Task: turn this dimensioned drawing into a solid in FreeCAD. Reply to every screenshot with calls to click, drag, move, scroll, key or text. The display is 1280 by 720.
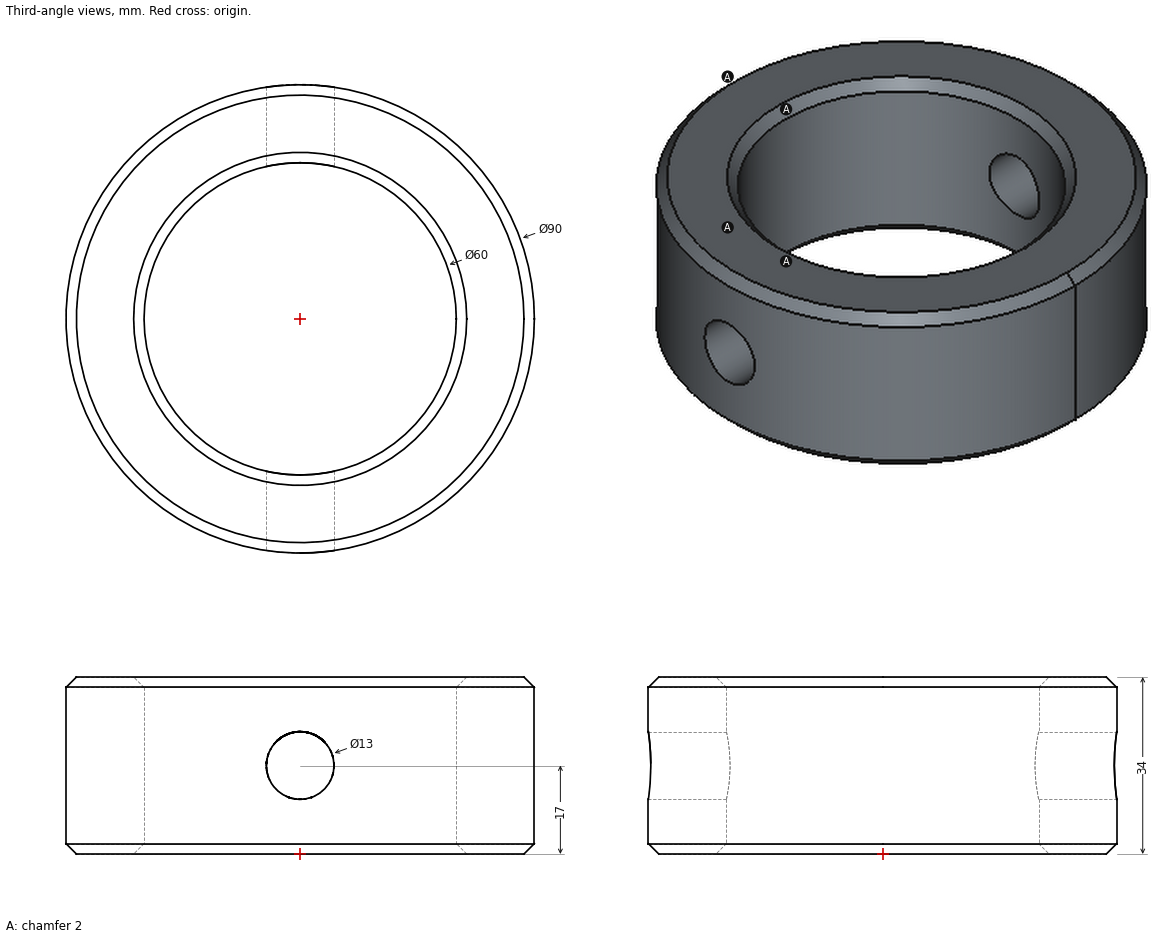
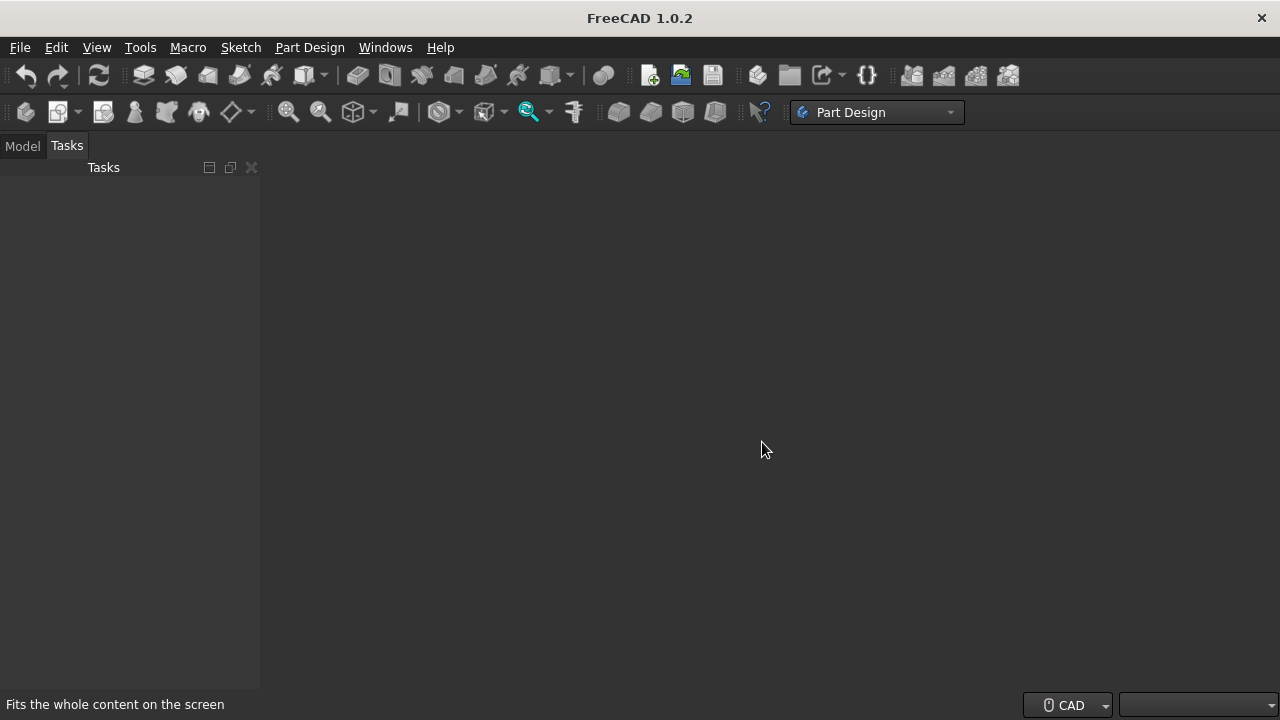
key(ctrl+n)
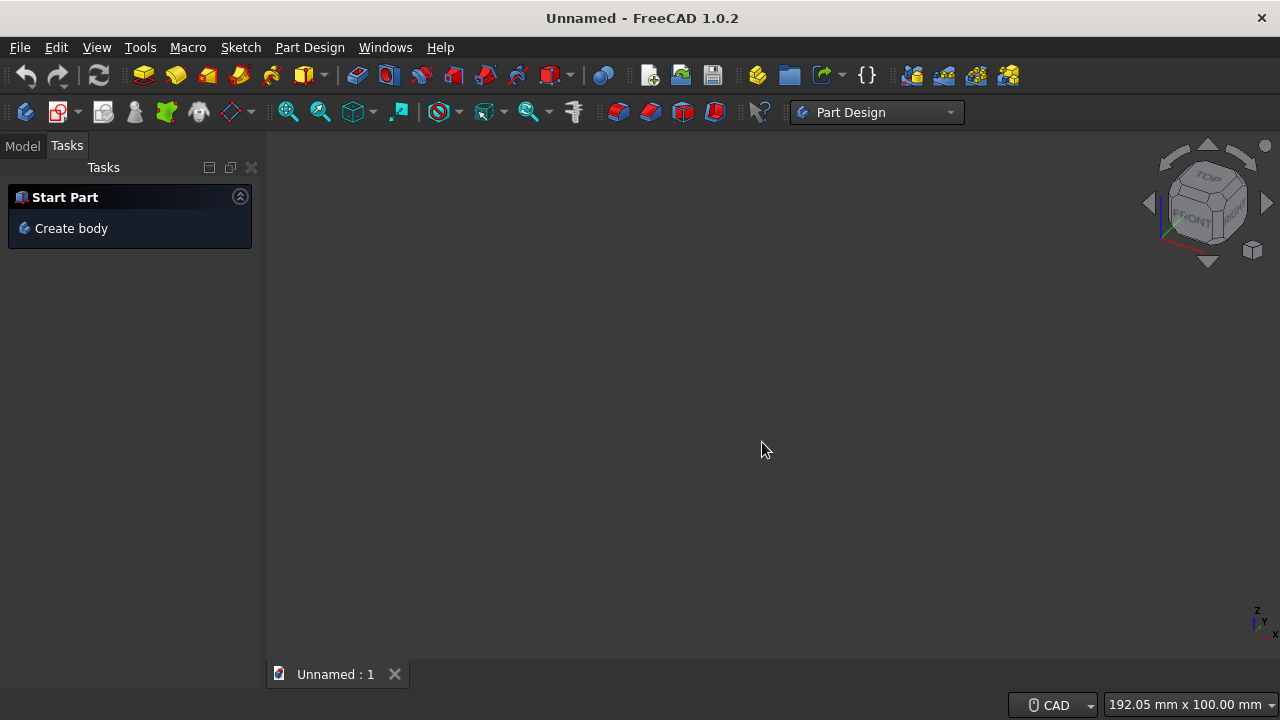
click(58, 112)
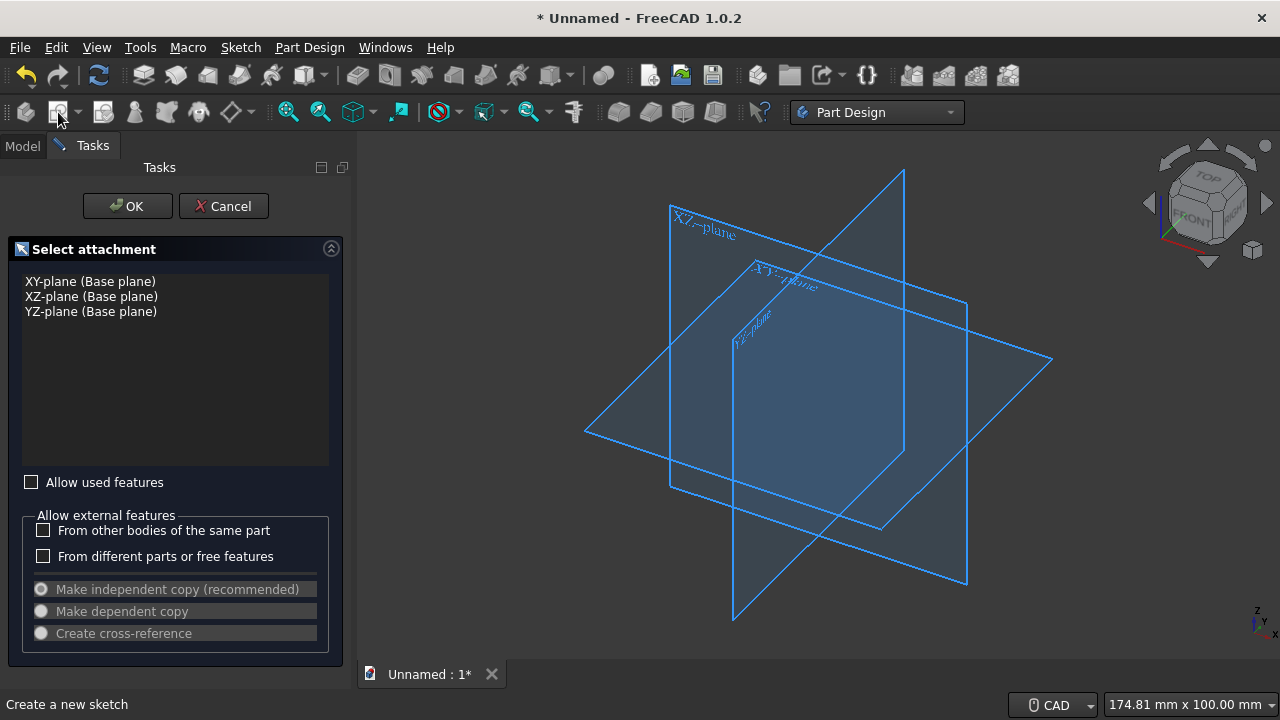
click(82, 282)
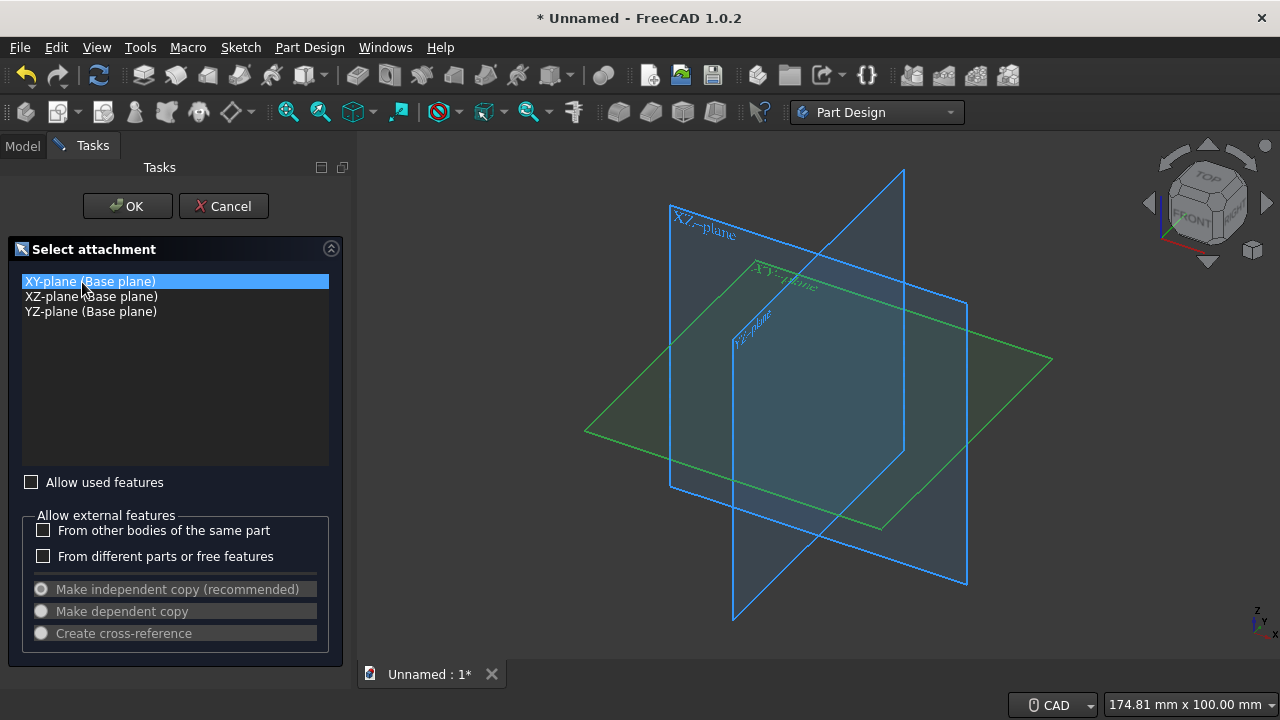
click(128, 206)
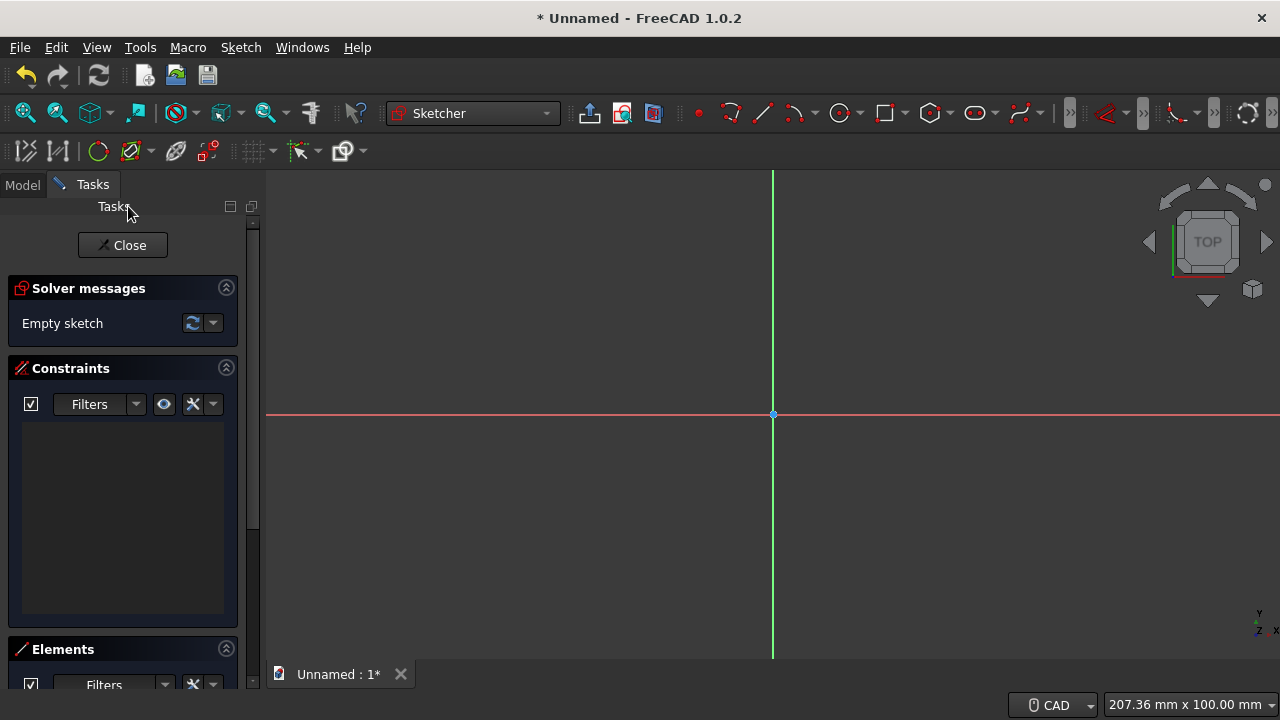
scroll(565, 414, down, 2)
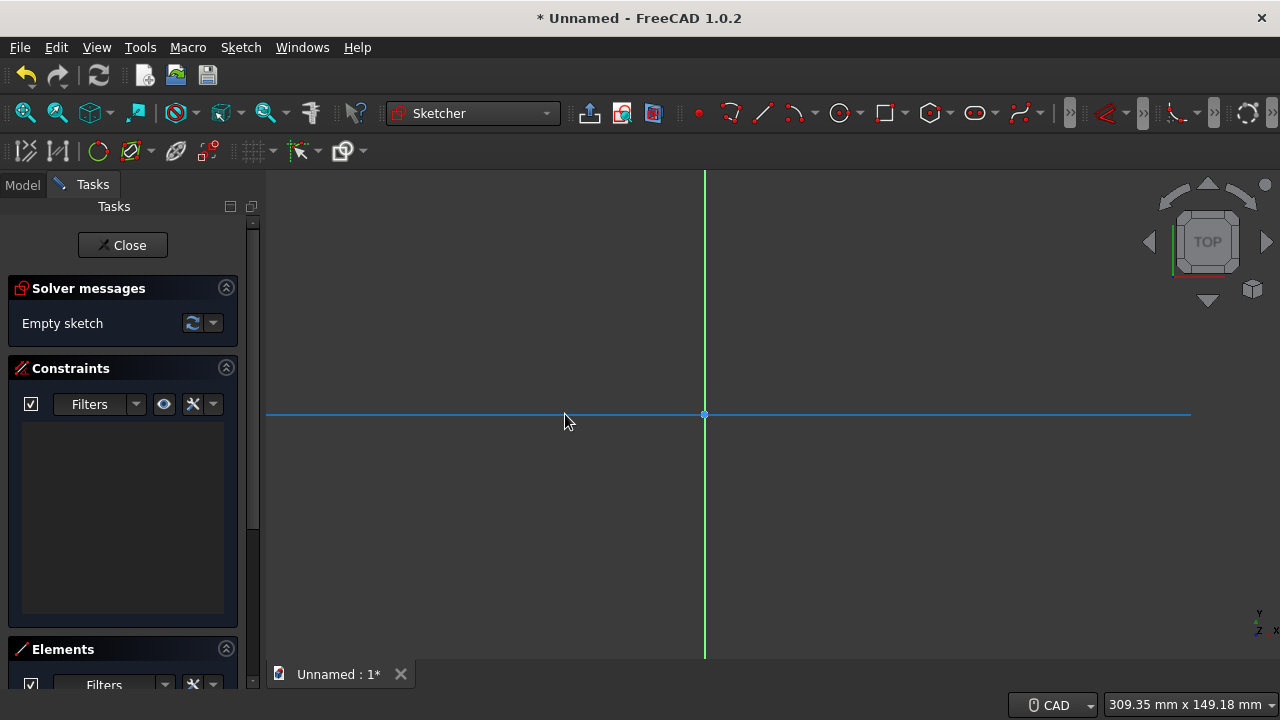
click(840, 114)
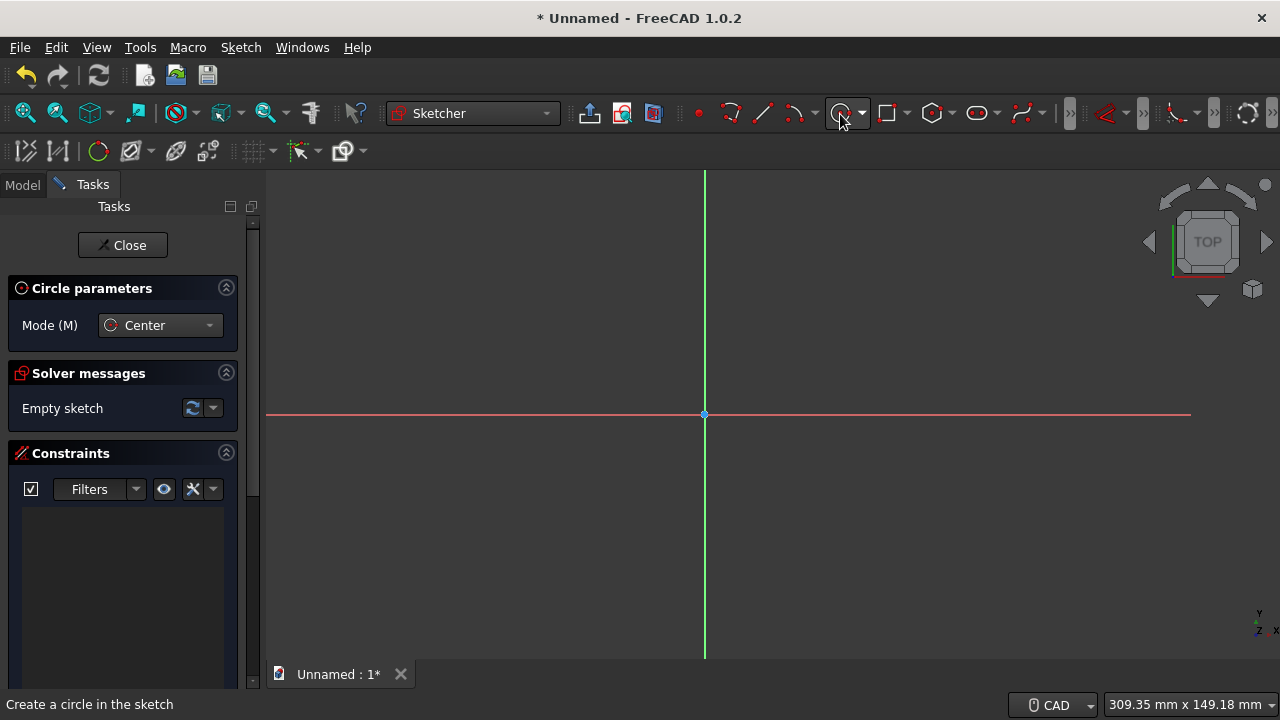
click(705, 414)
move(809, 310)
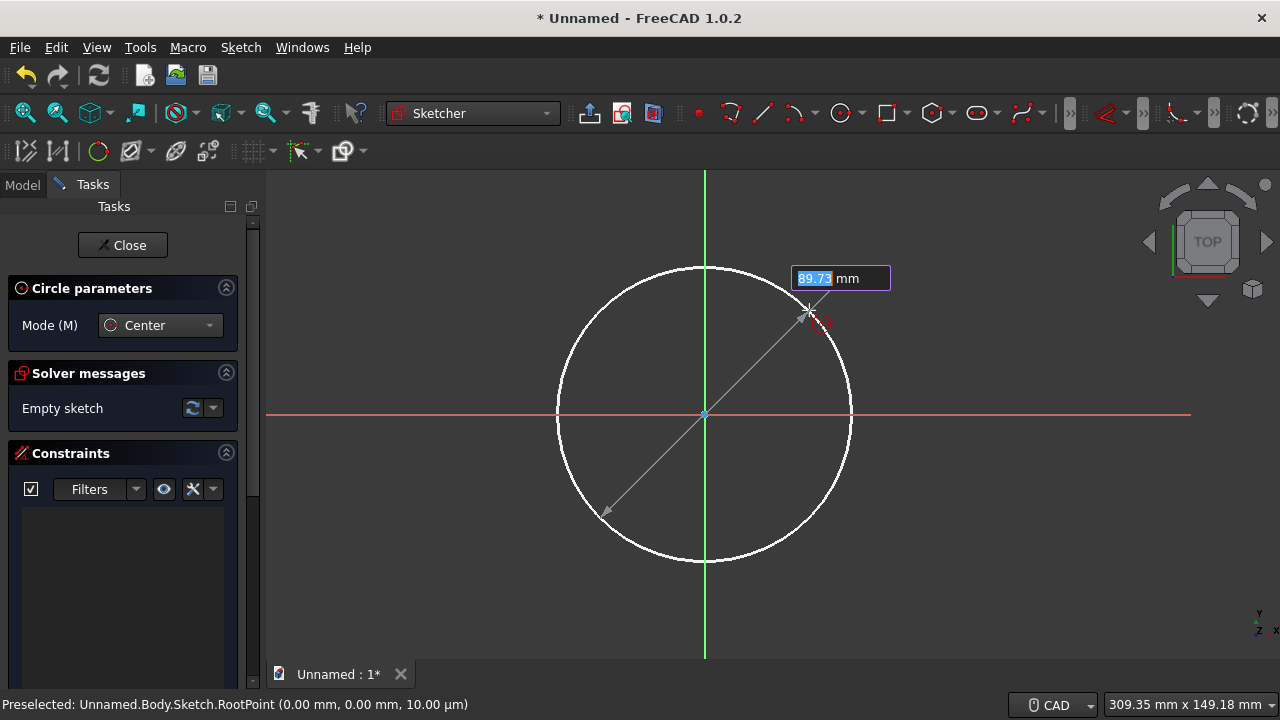
text(90)
key(Return)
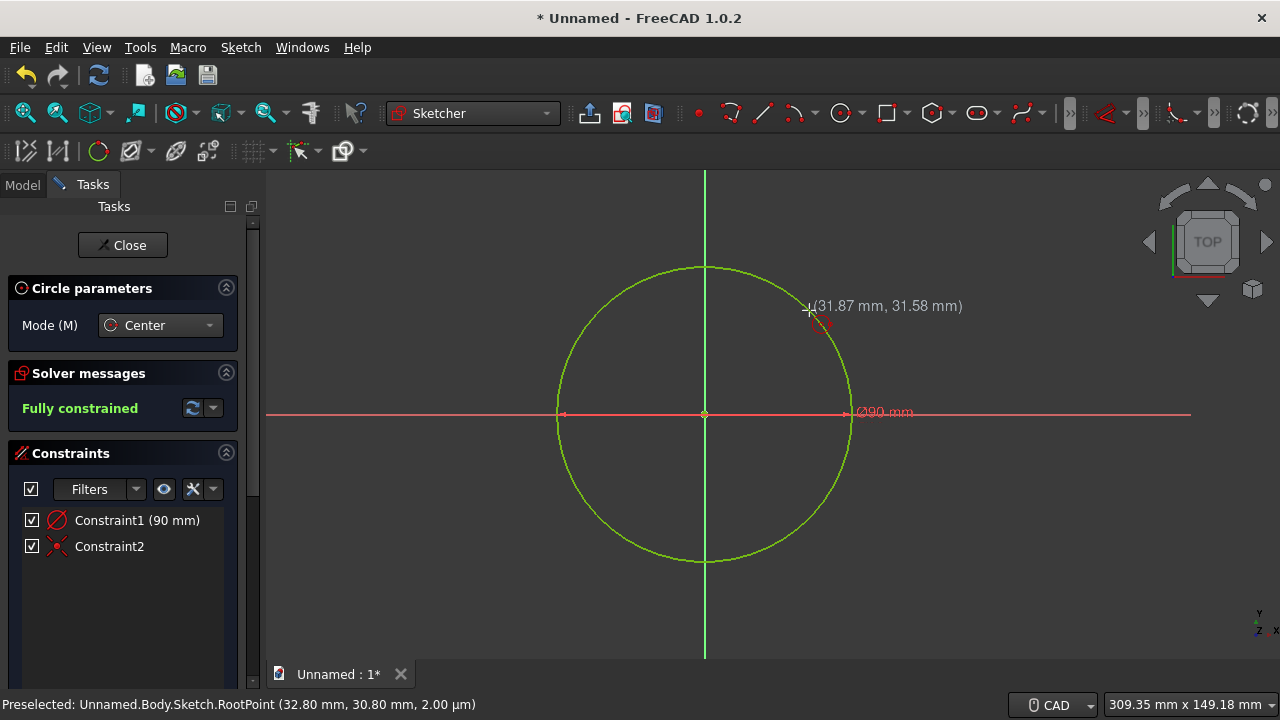
click(705, 414)
move(774, 345)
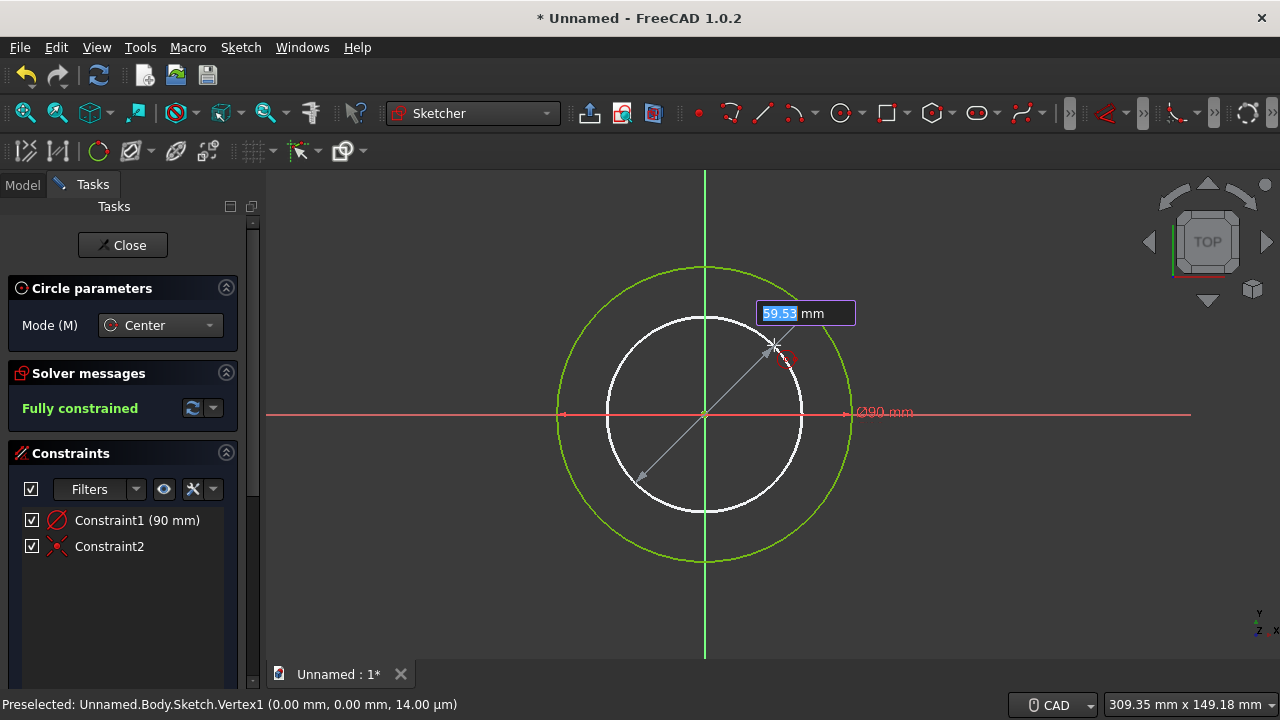
text(60)
key(Return)
key(Escape)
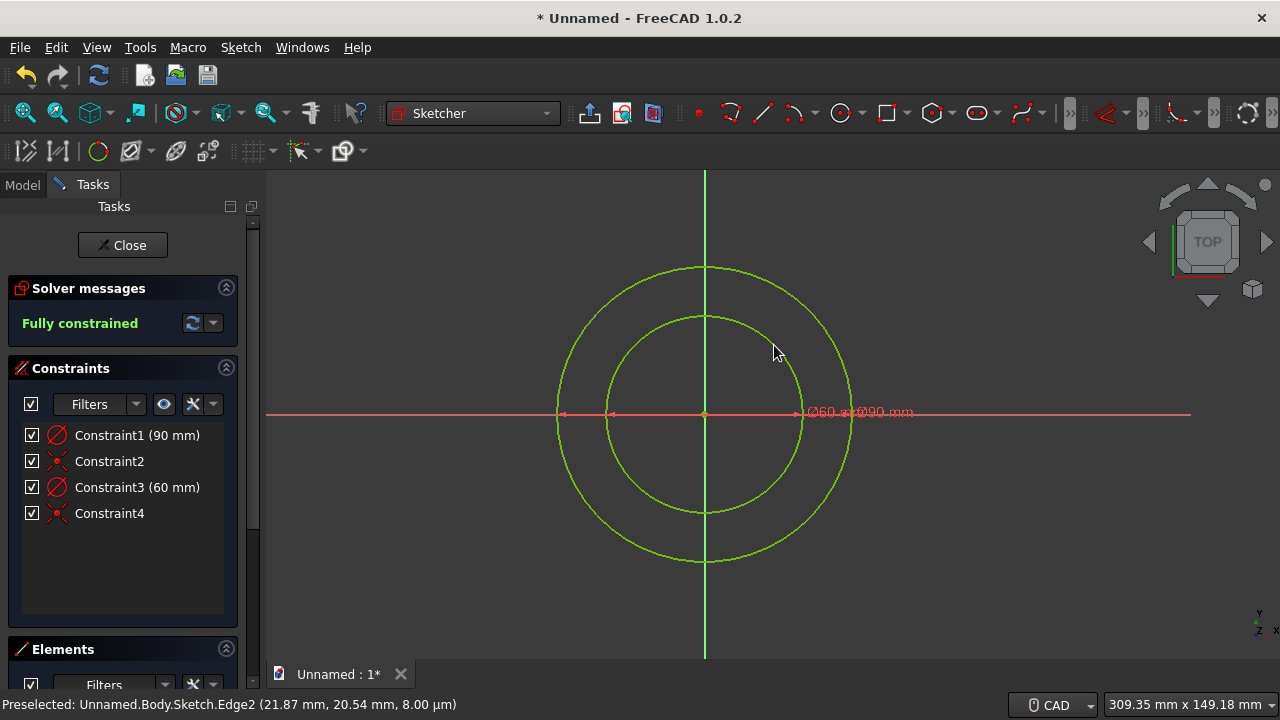
click(123, 245)